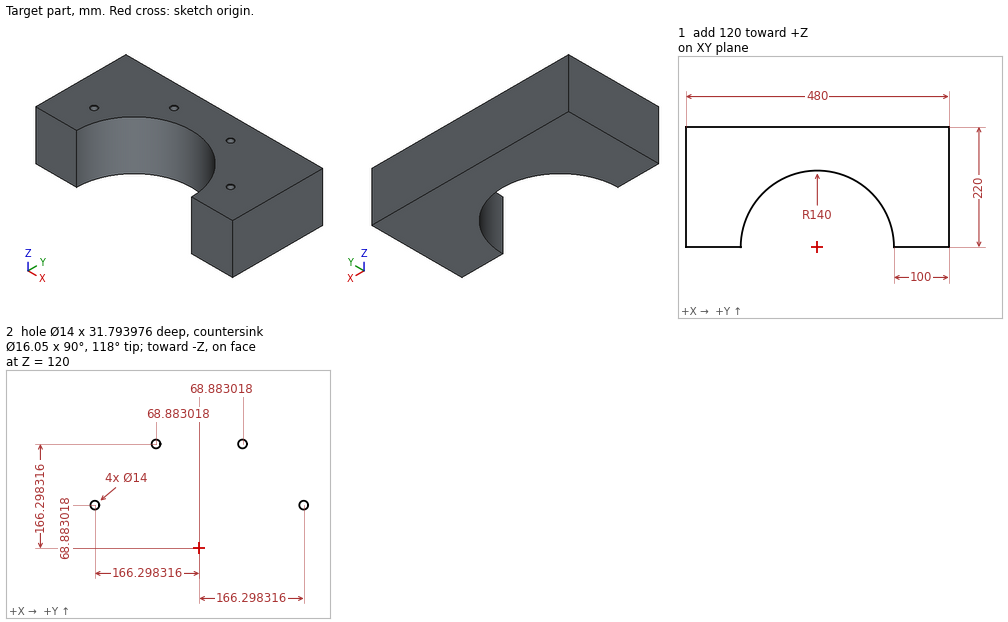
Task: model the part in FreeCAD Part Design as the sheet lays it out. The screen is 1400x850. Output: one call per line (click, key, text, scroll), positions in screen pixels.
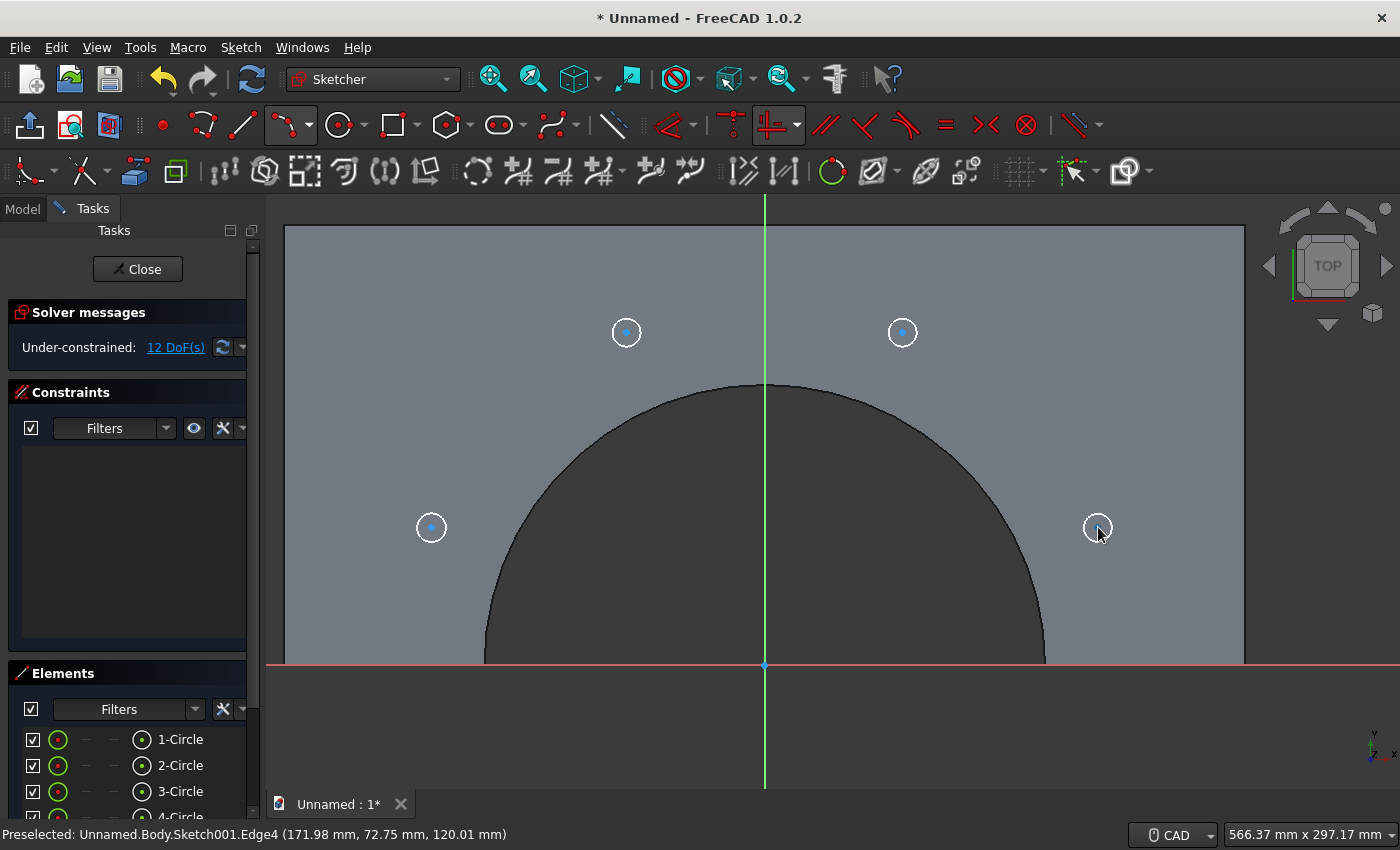
click(442, 518)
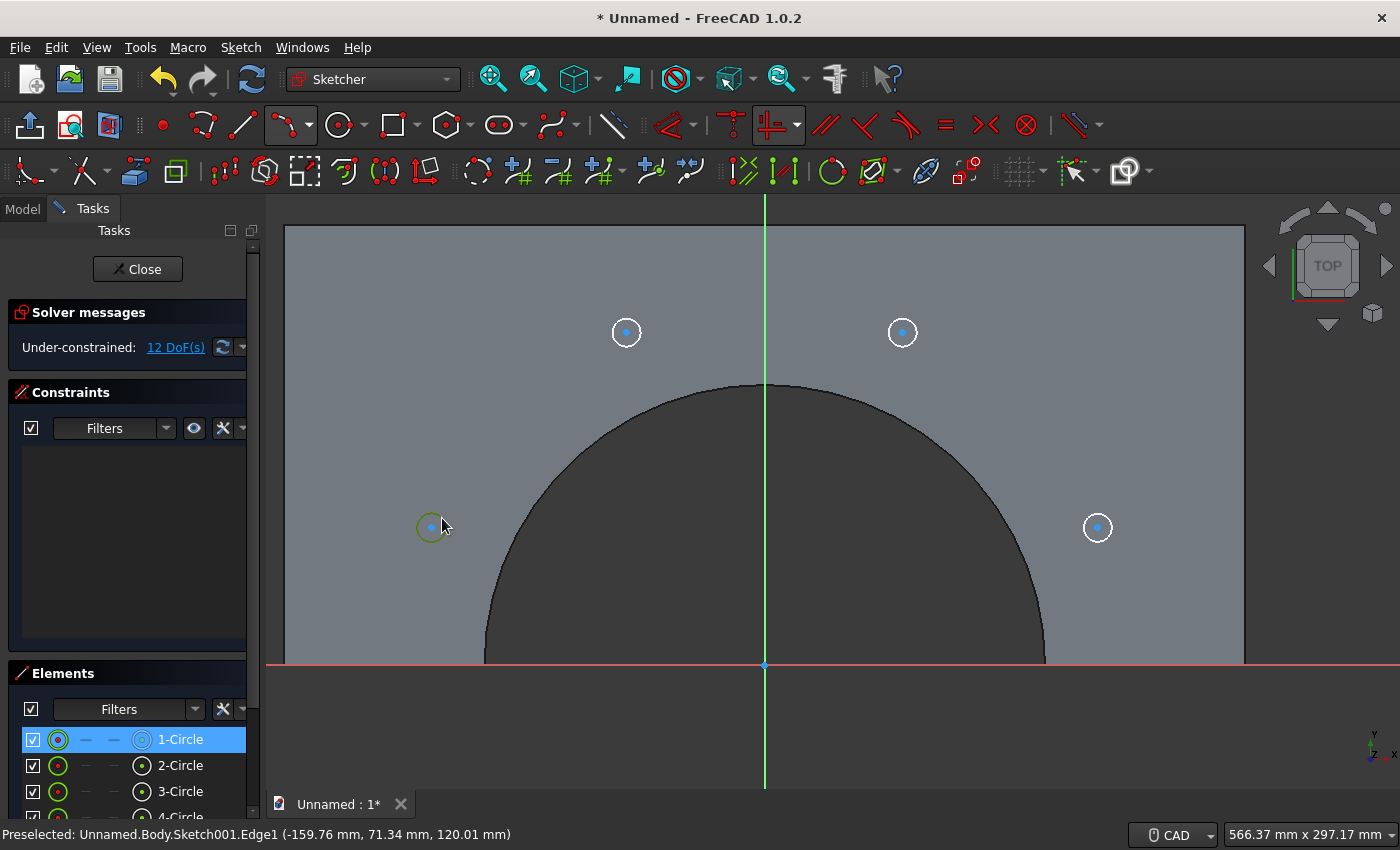
click(636, 323)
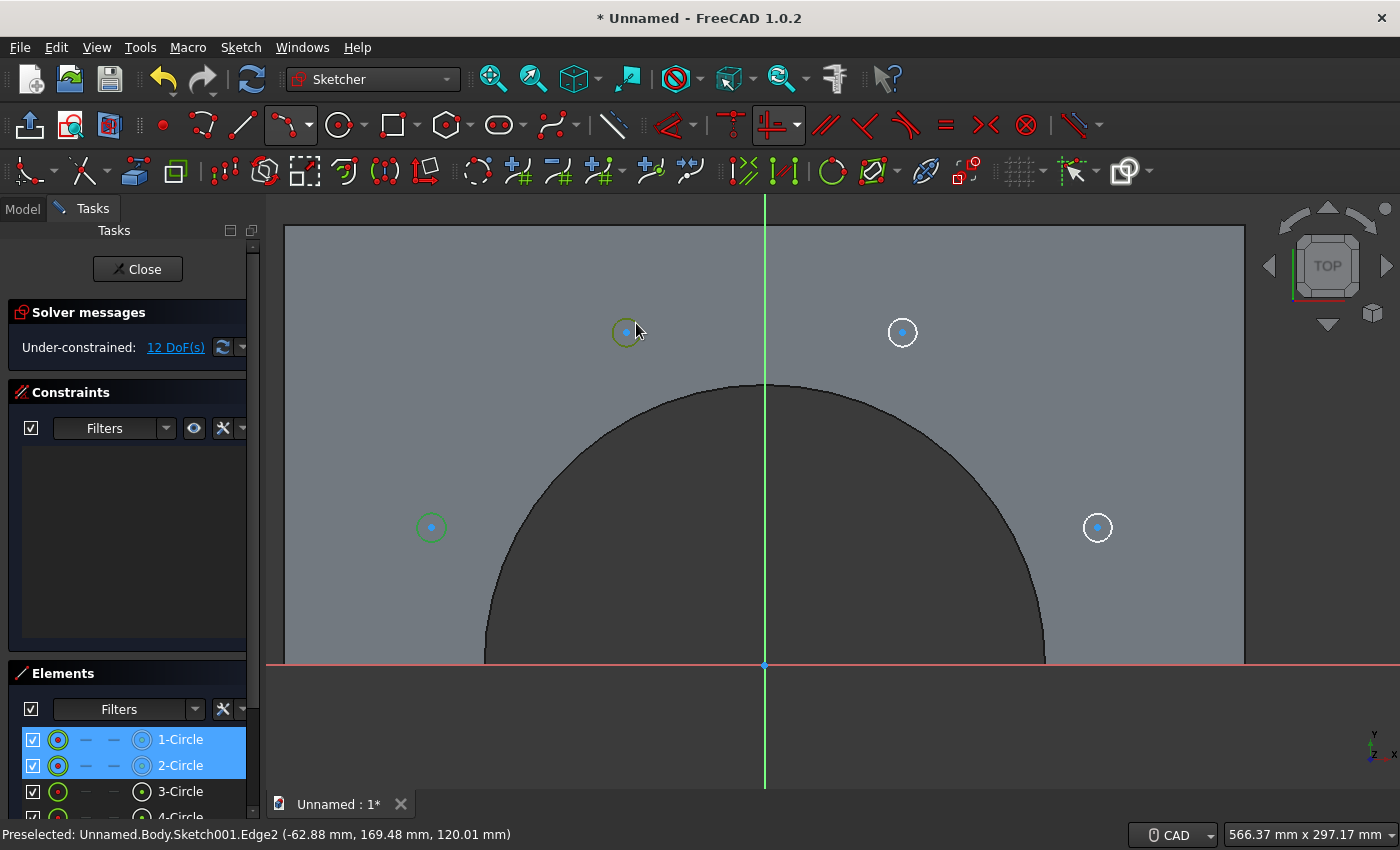
click(912, 323)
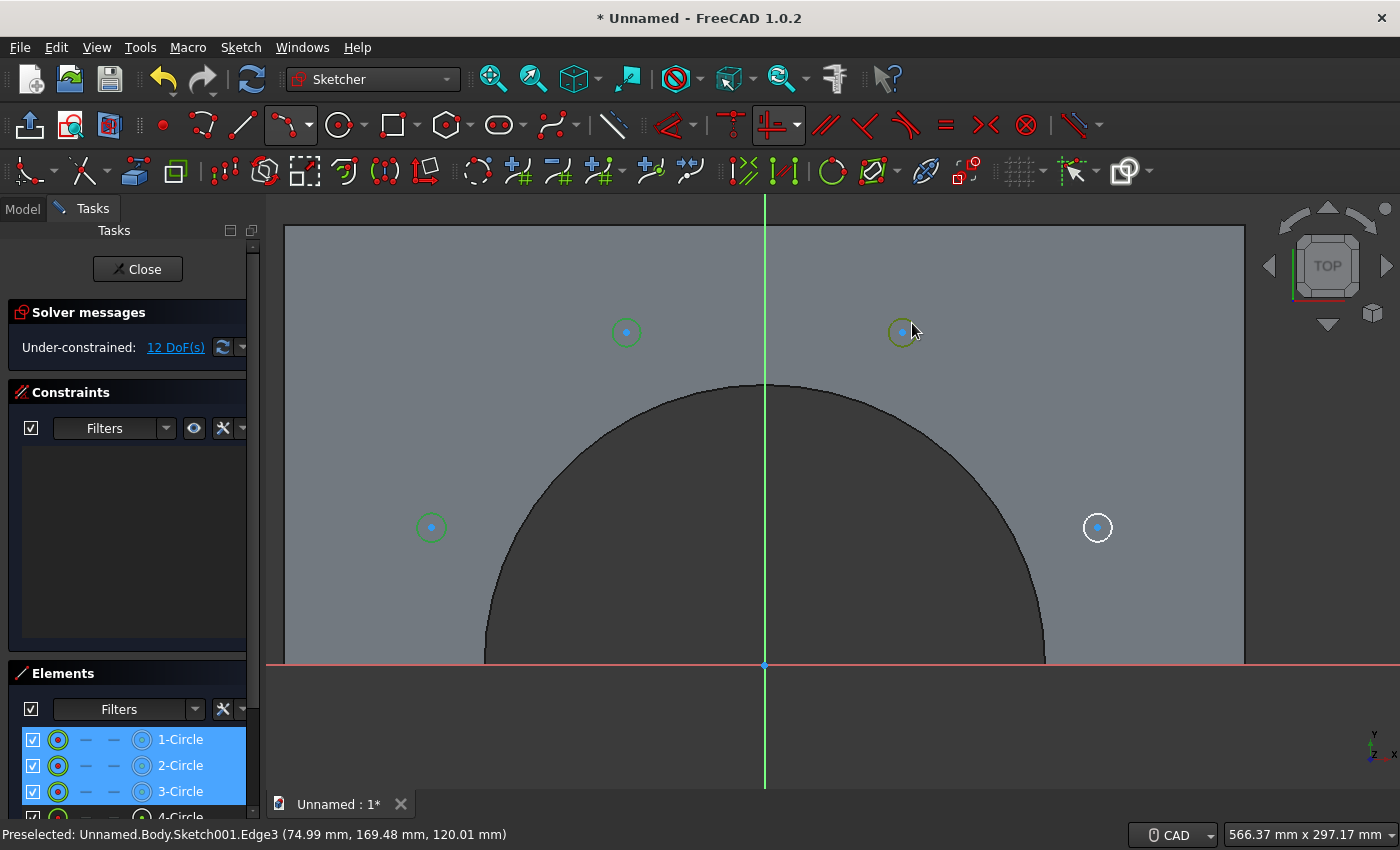
click(1108, 518)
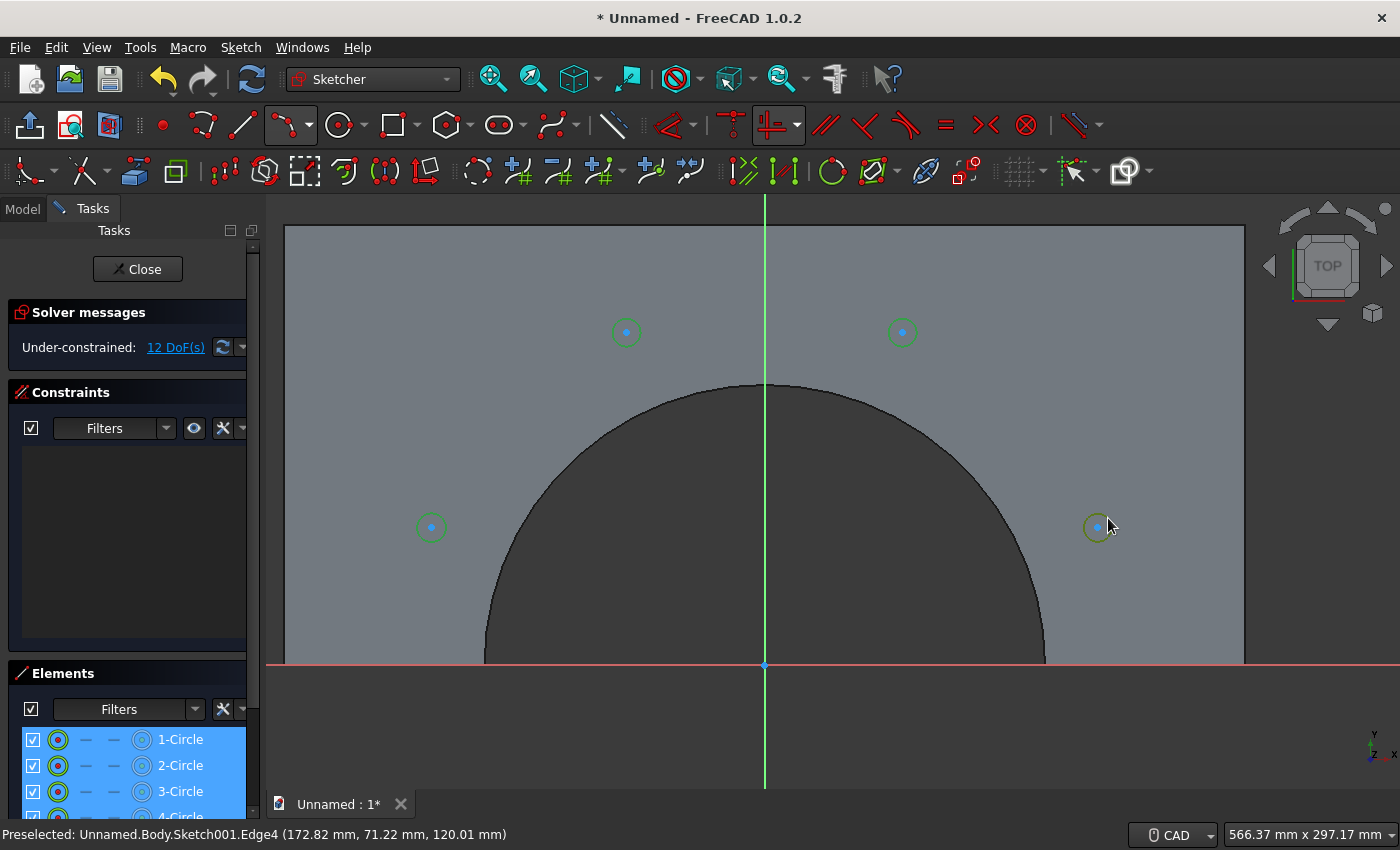
click(946, 126)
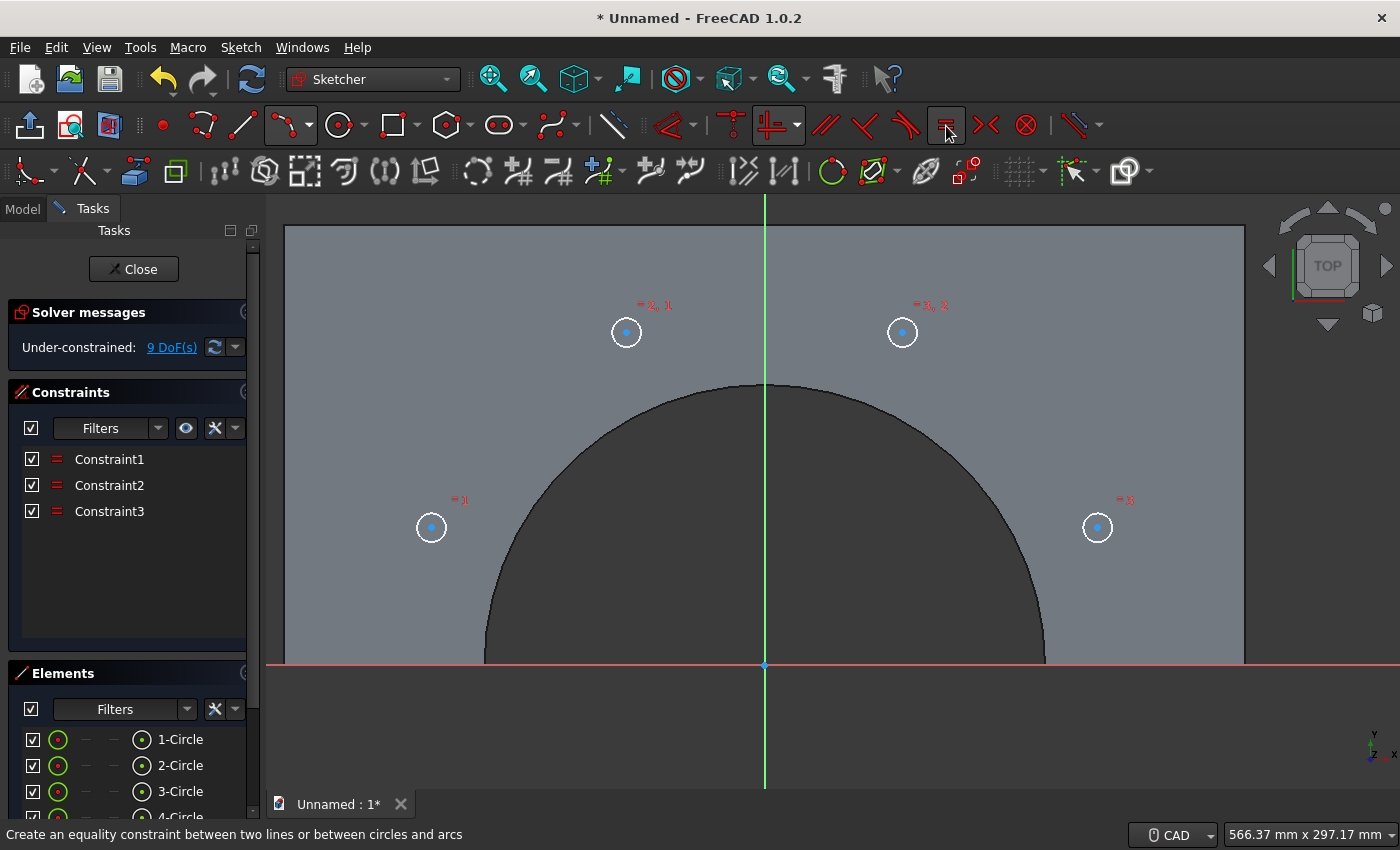
click(627, 333)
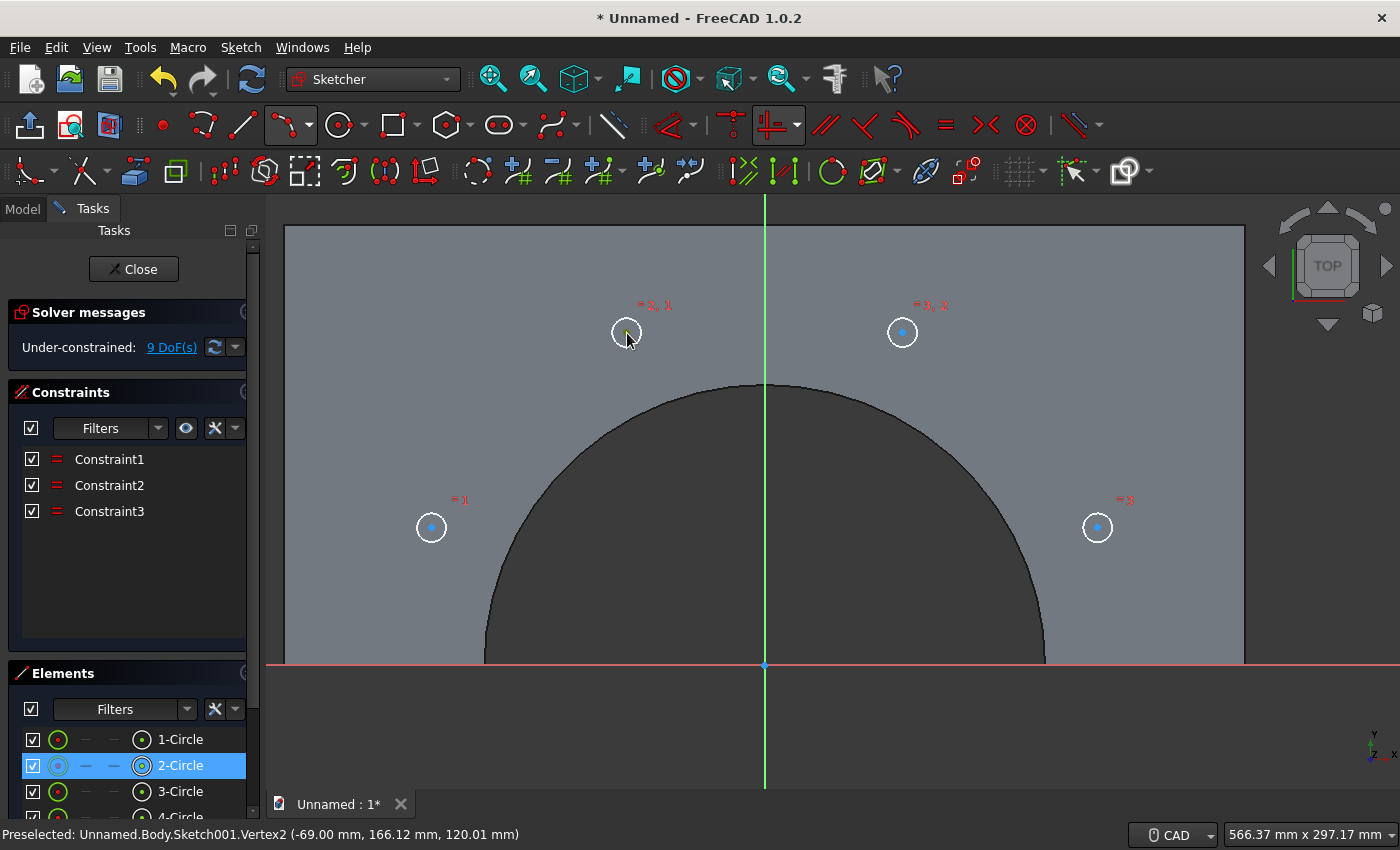
click(903, 333)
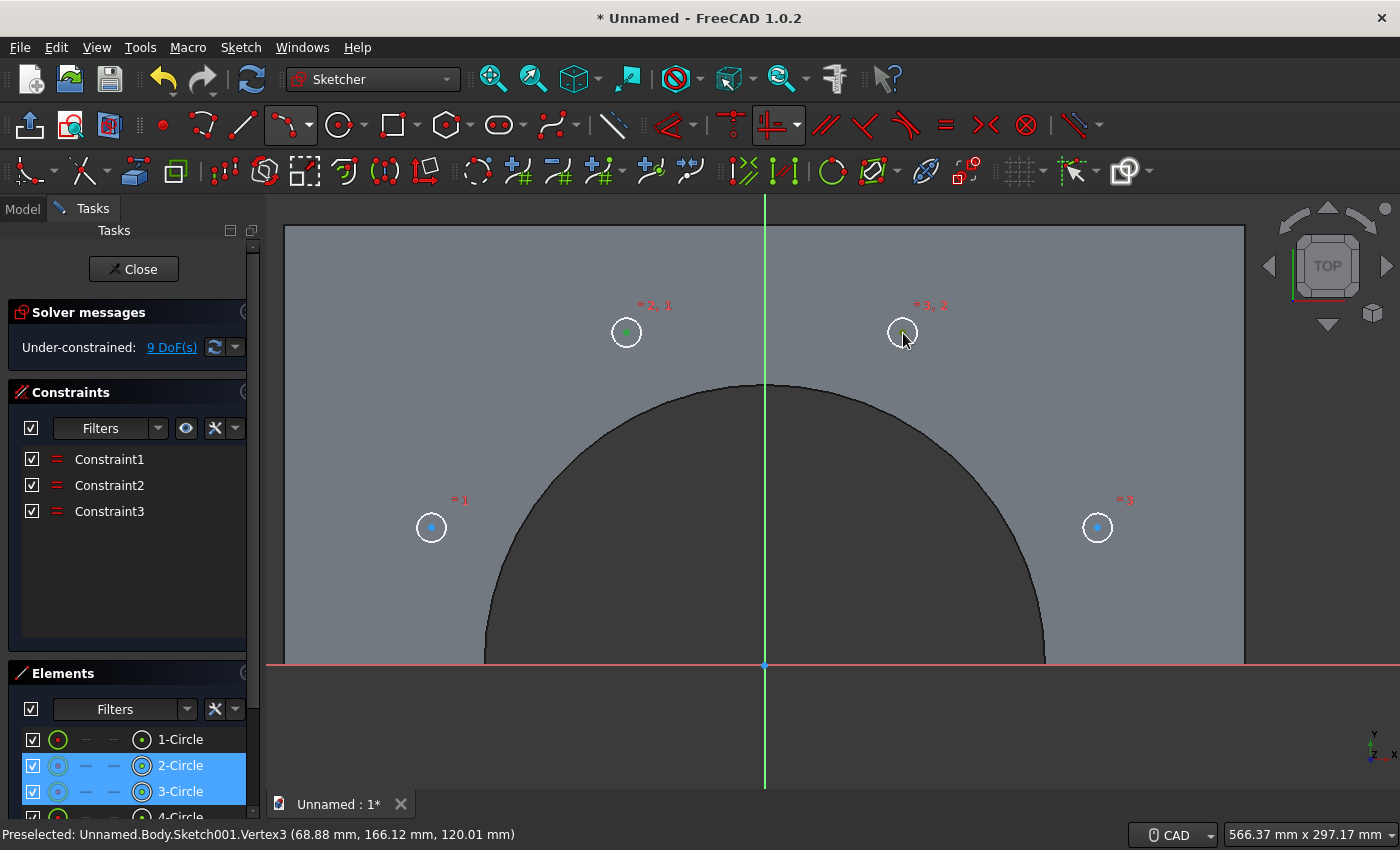
click(800, 126)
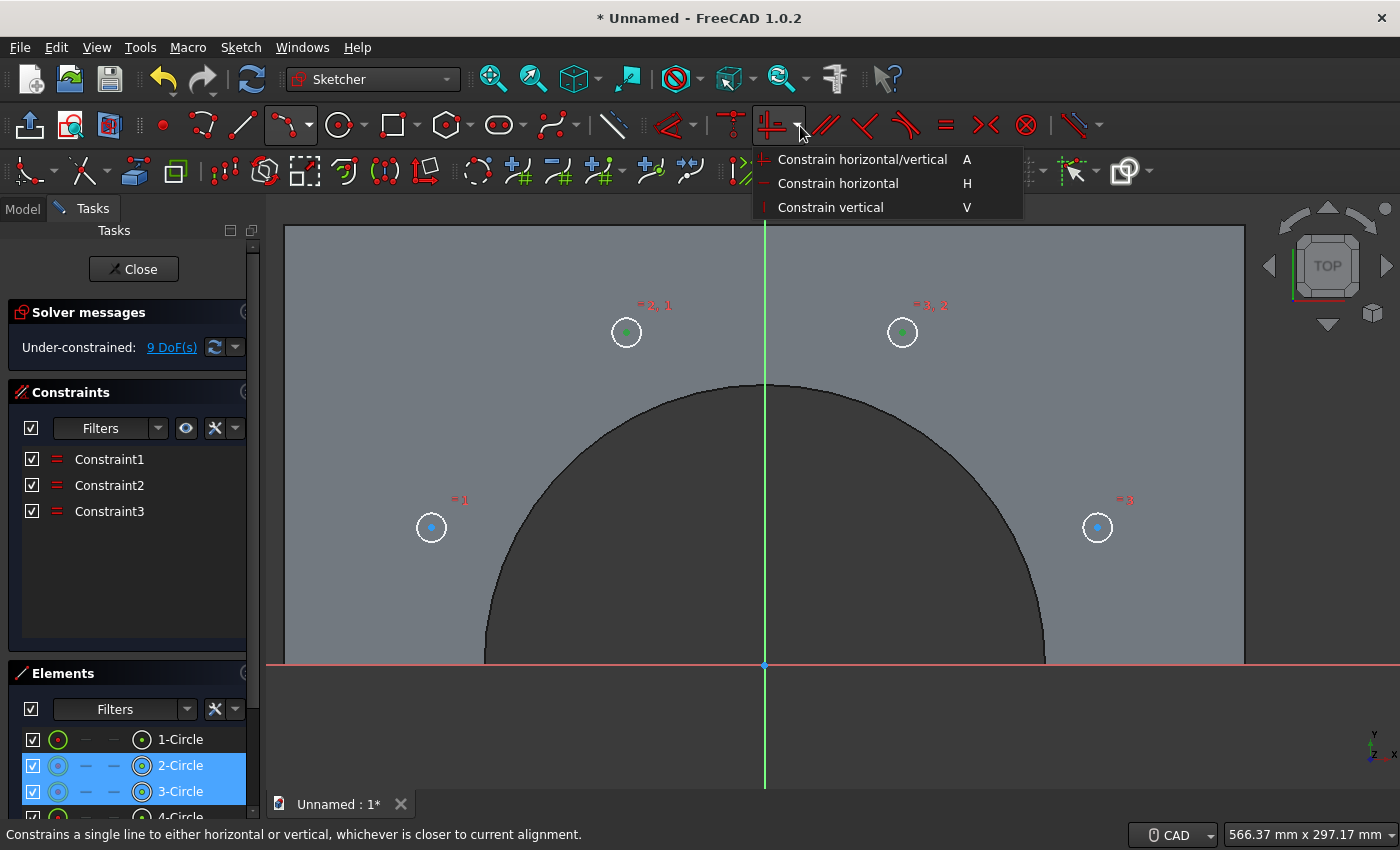
click(888, 183)